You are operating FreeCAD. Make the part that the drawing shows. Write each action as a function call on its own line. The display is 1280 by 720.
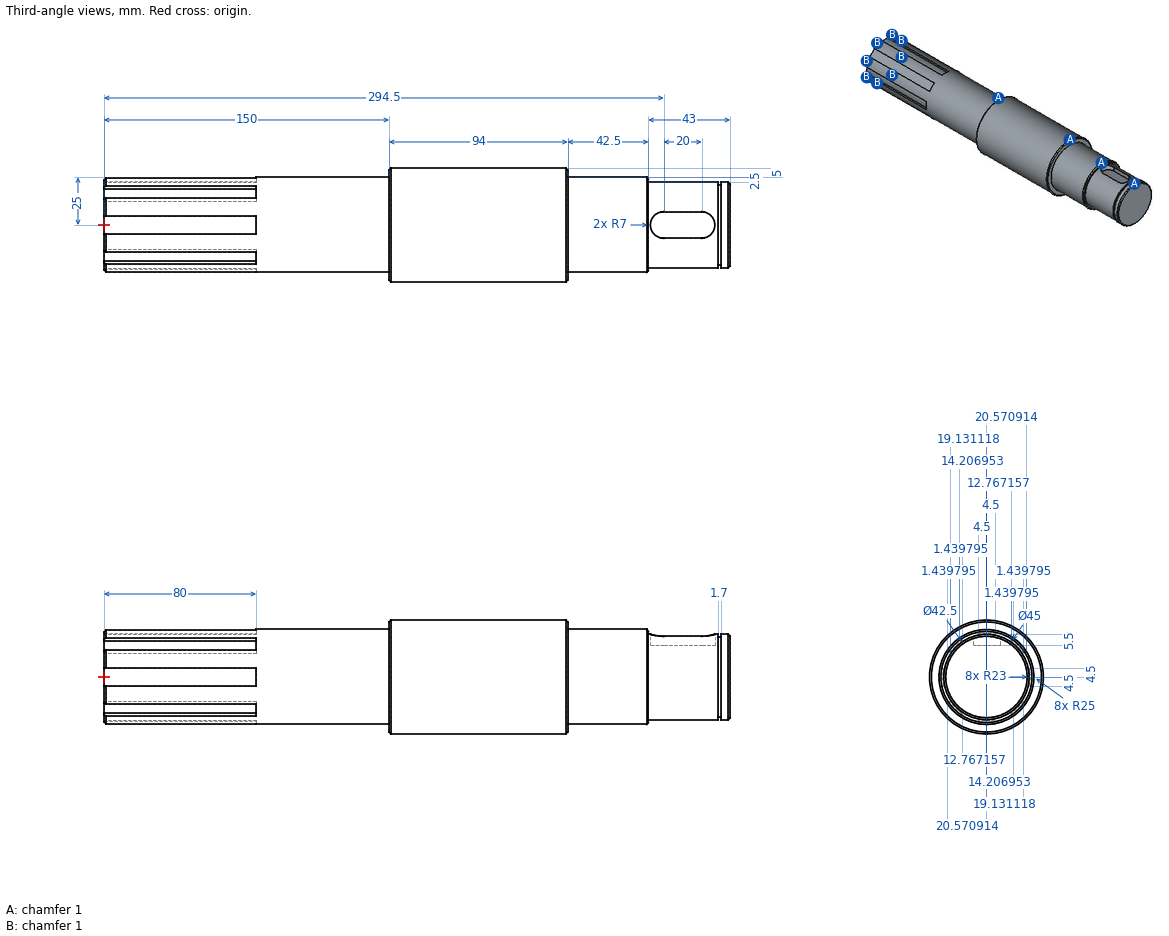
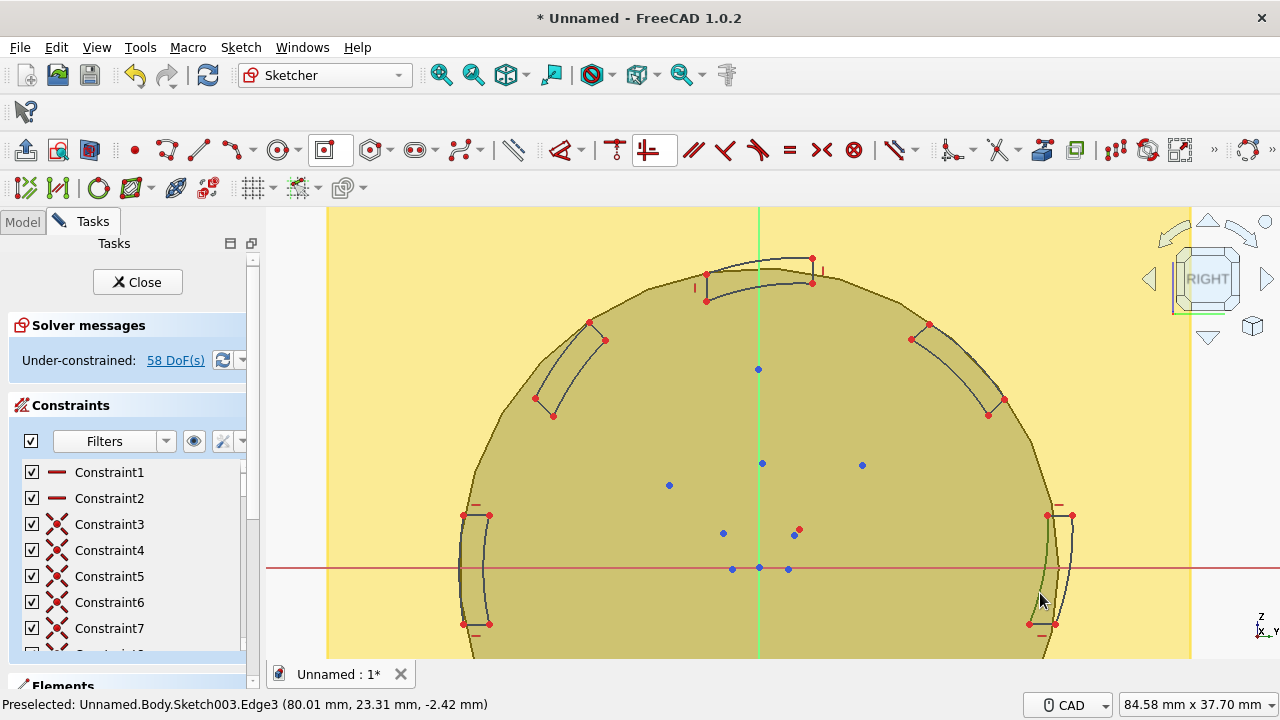
click(460, 548)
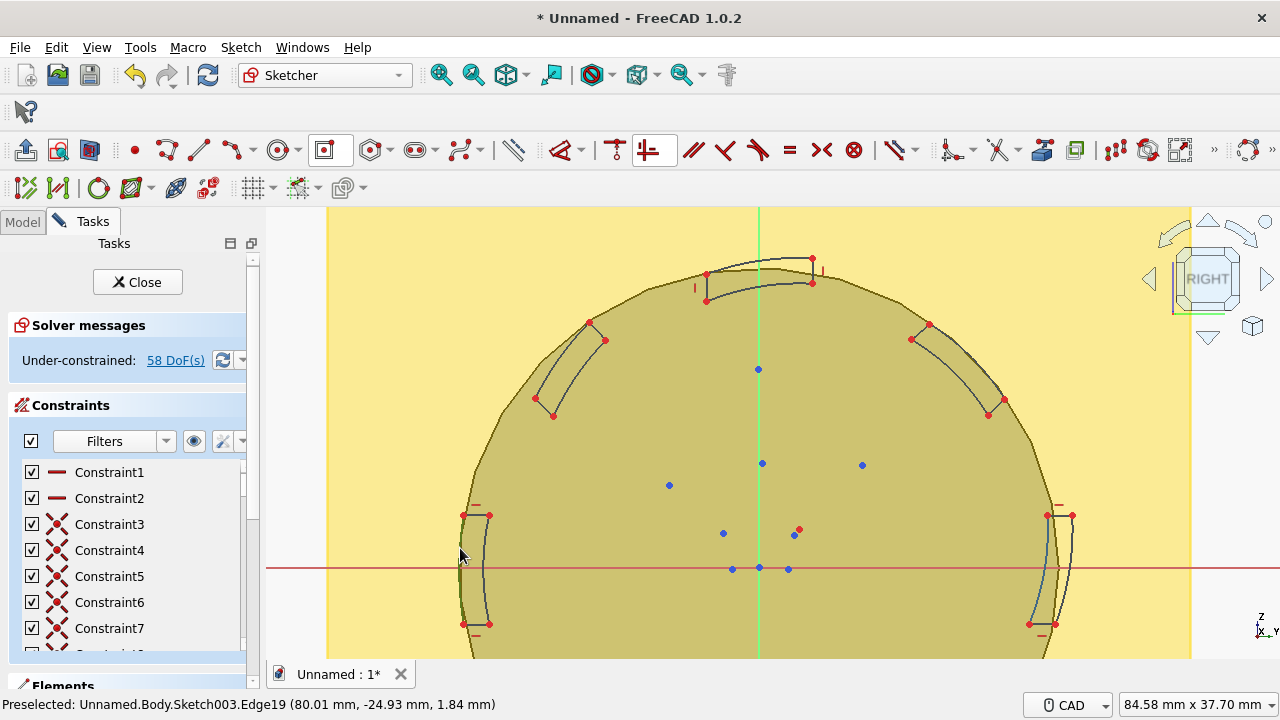
click(616, 150)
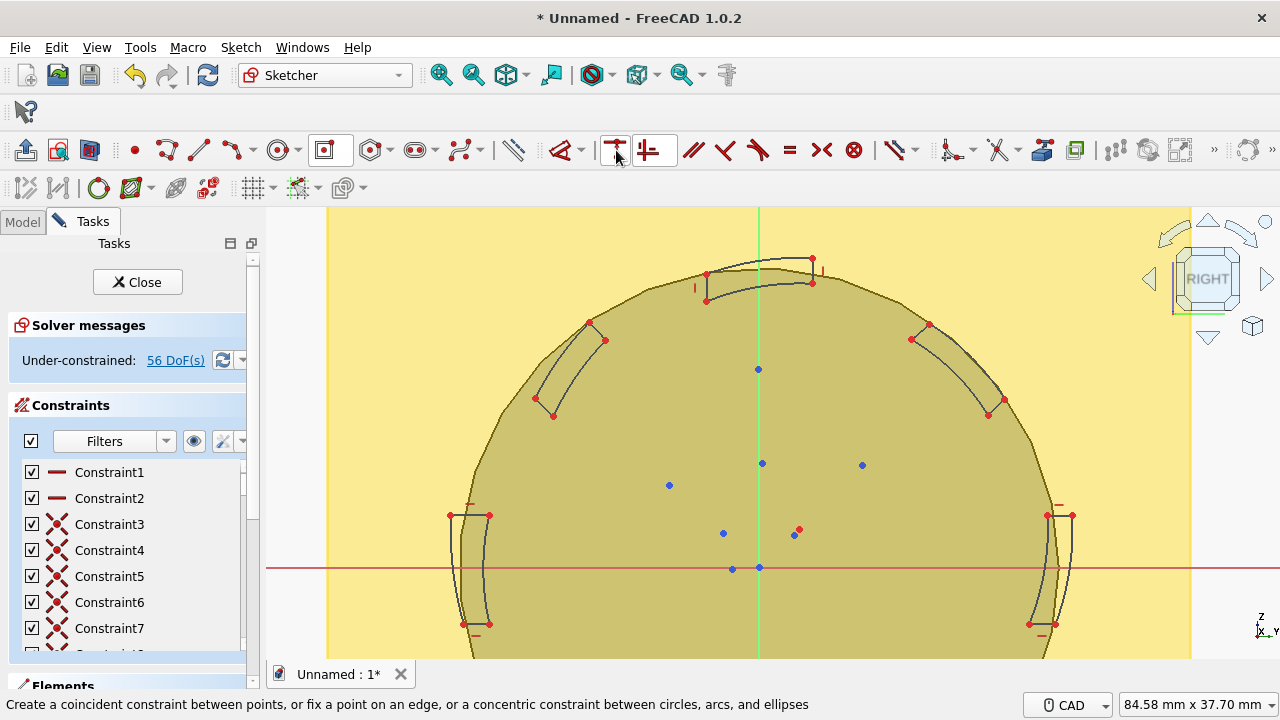
click(1040, 593)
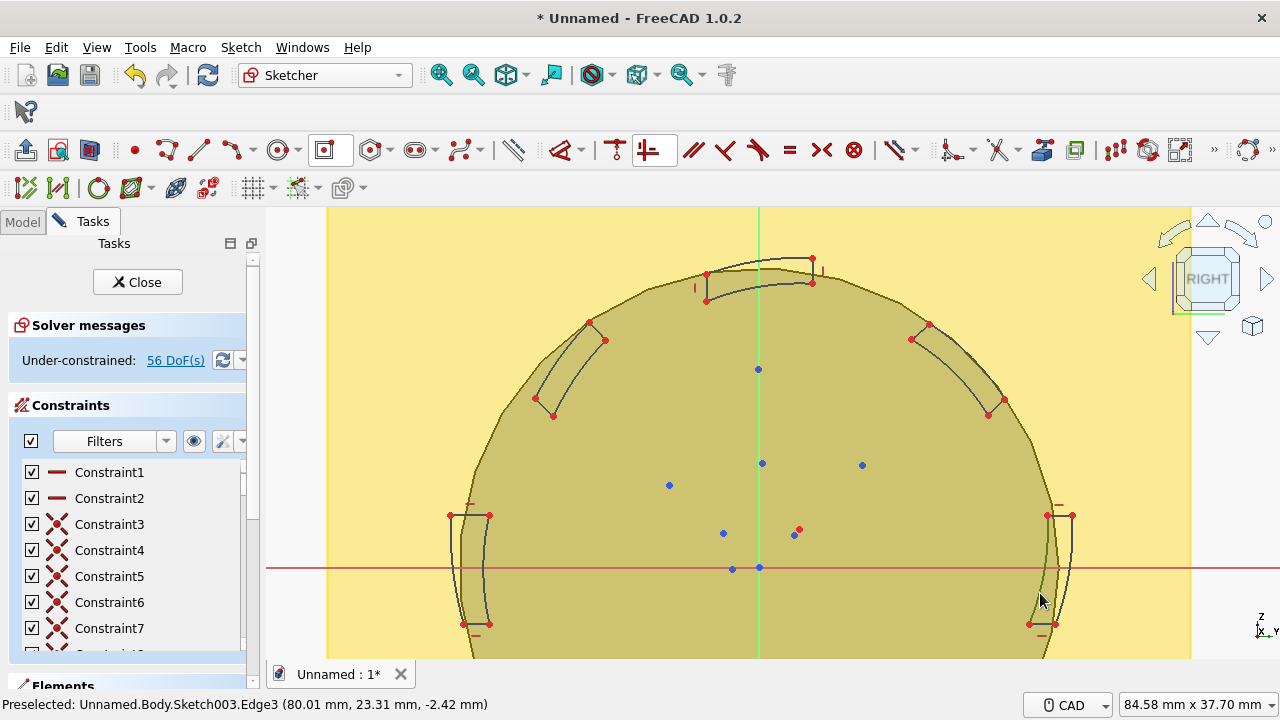
click(484, 548)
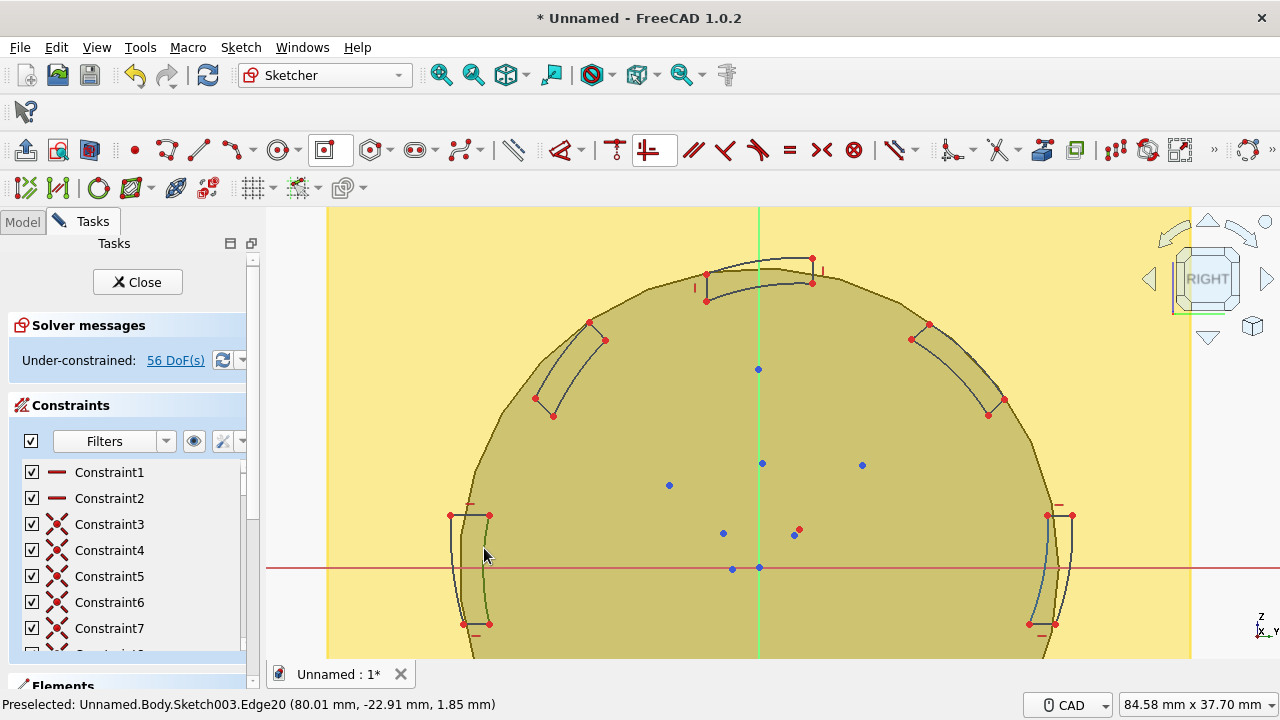
click(616, 150)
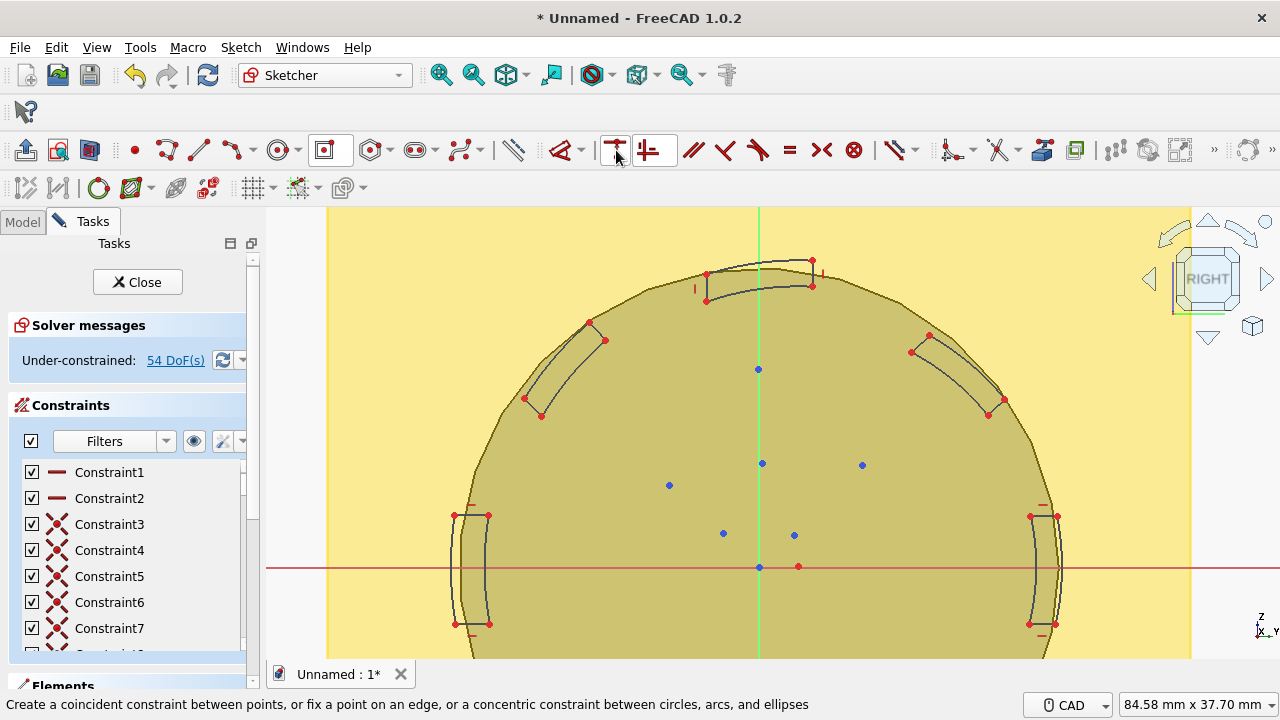
click(1035, 592)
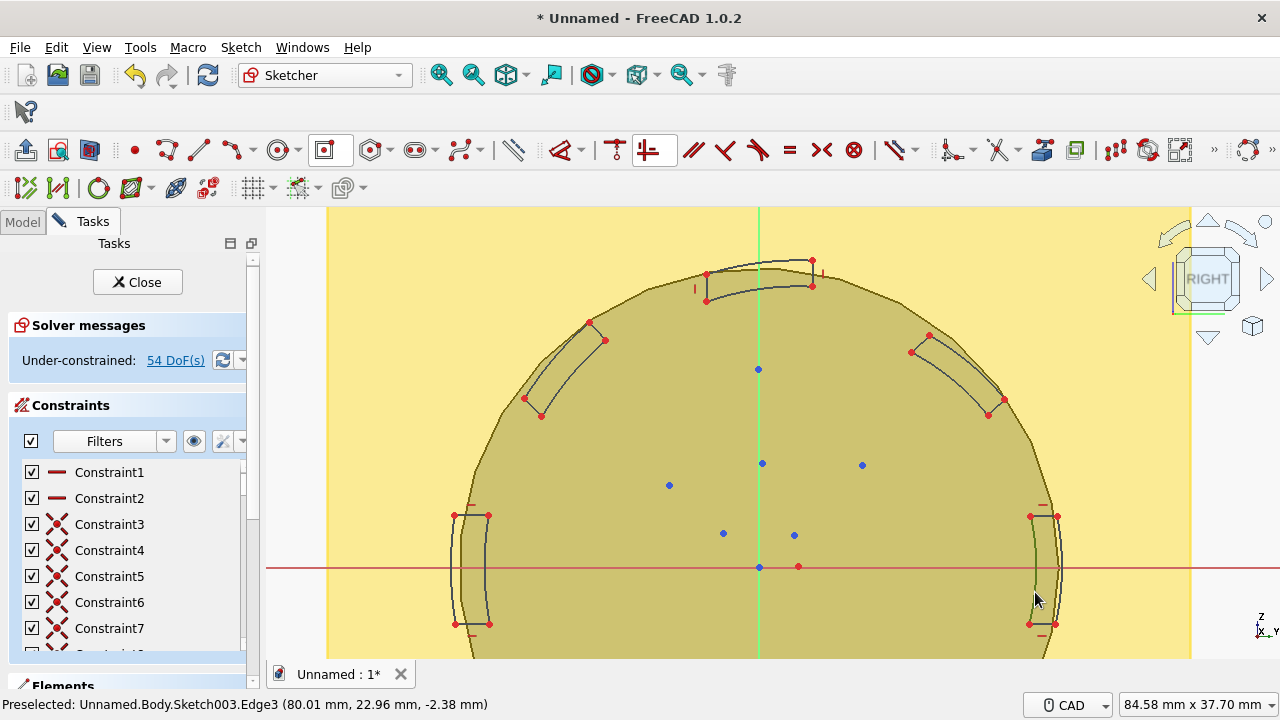
scroll(660, 323, down, 4)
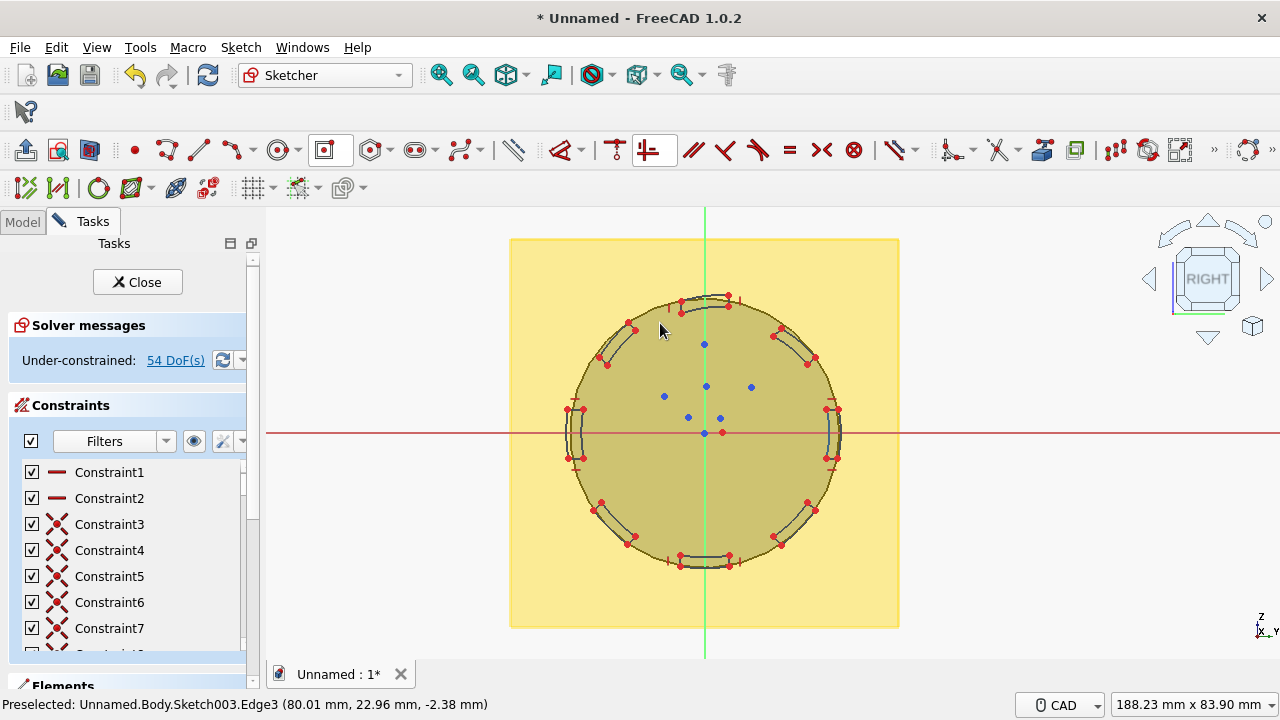
scroll(603, 522, up, 2)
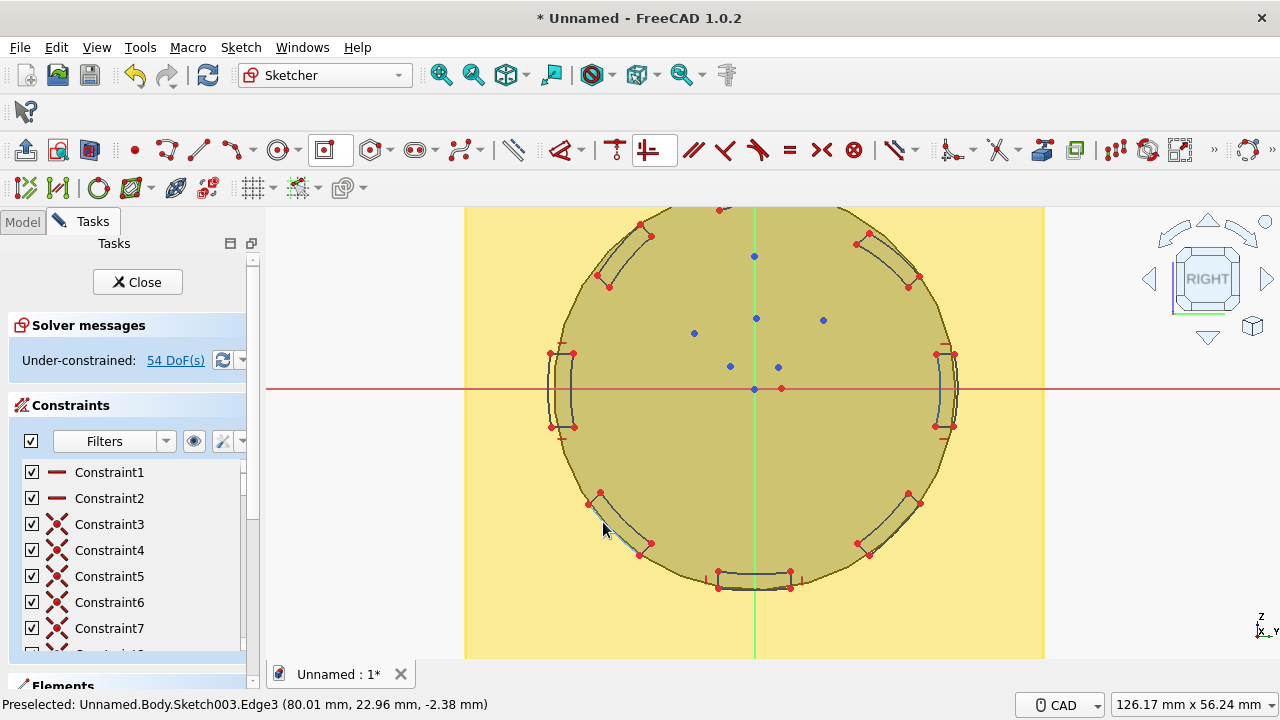
click(603, 521)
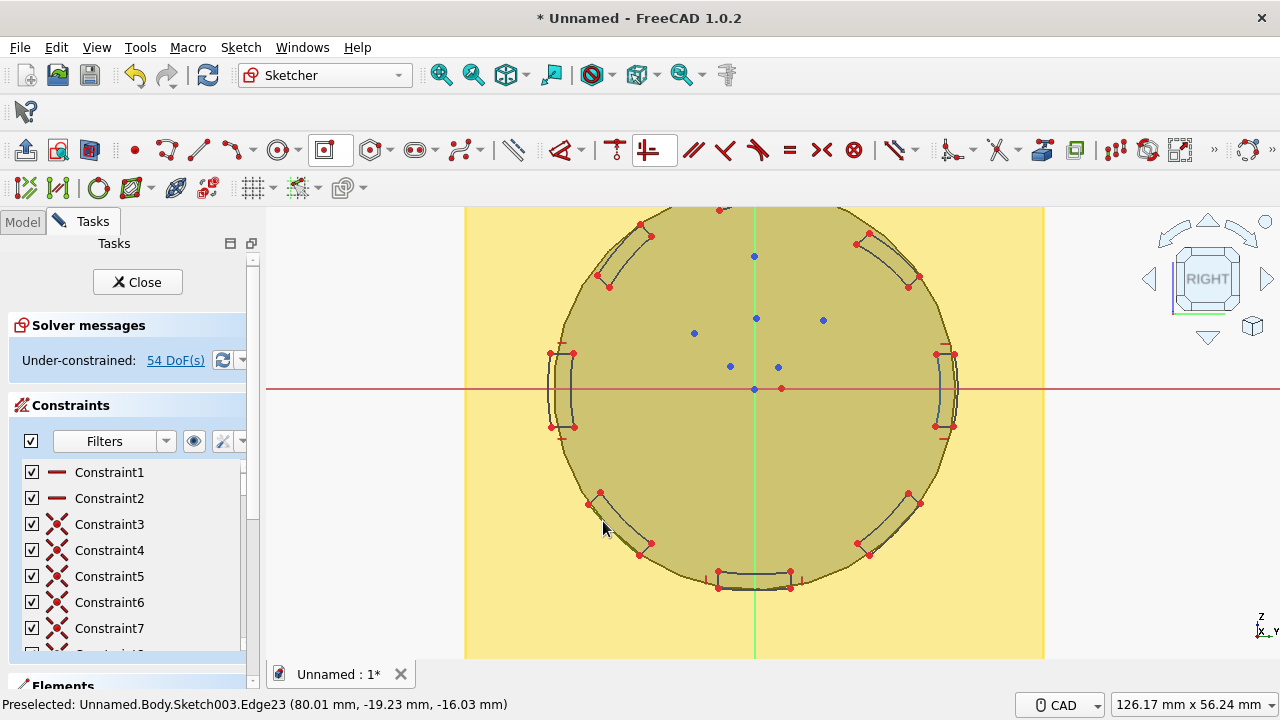
click(616, 150)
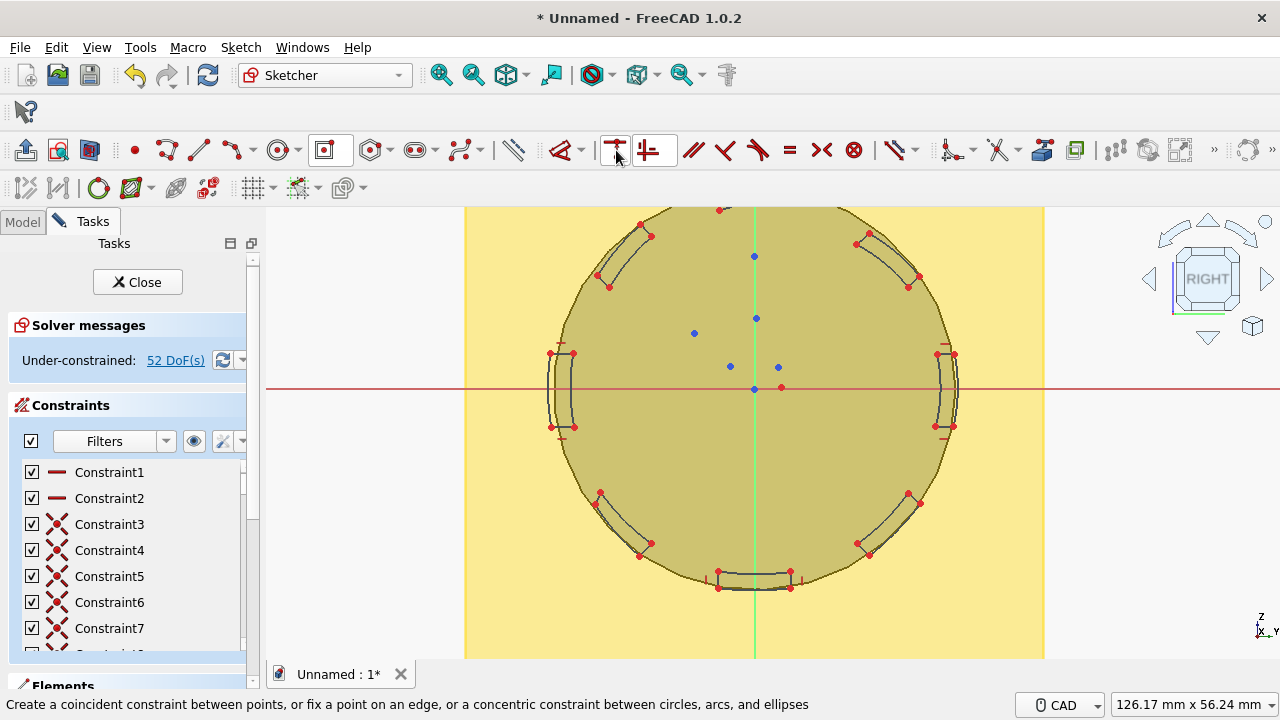
click(940, 405)